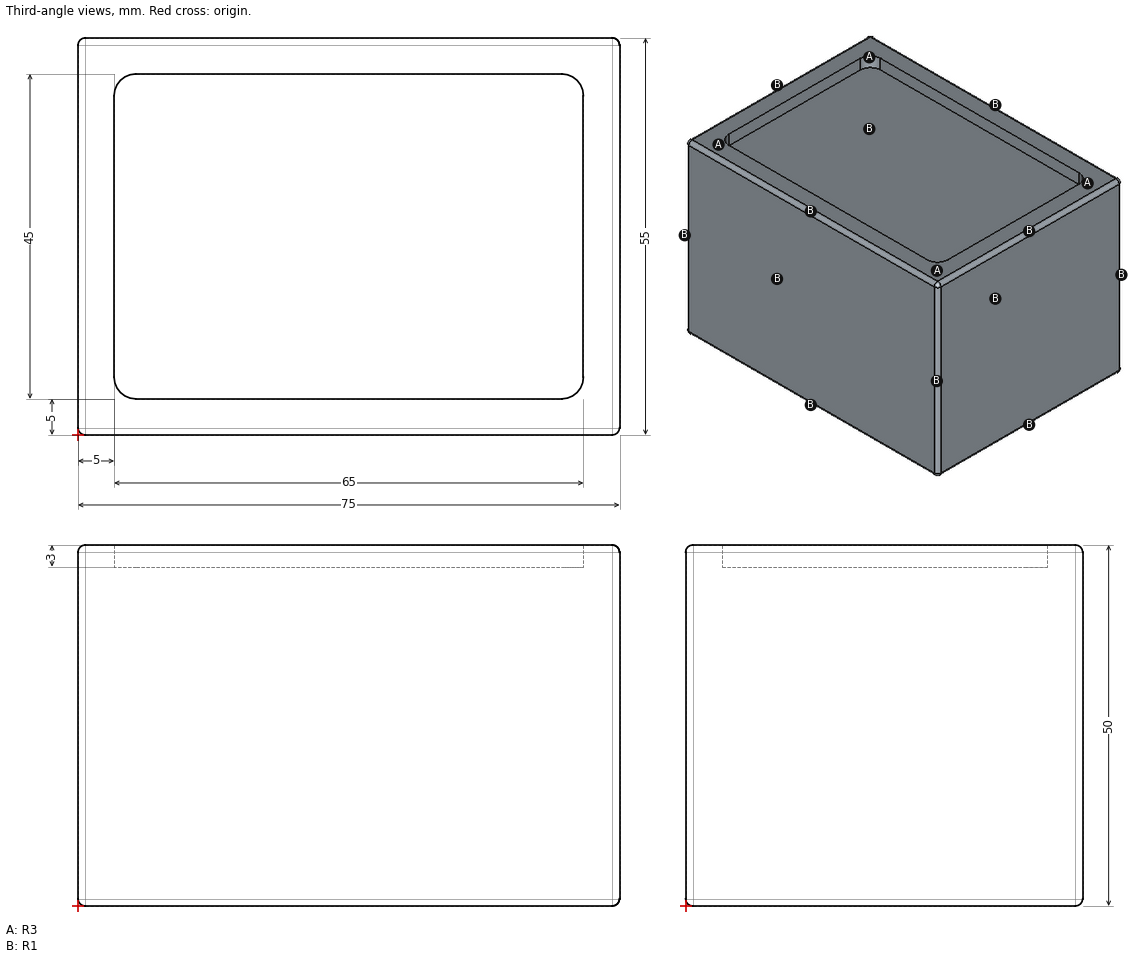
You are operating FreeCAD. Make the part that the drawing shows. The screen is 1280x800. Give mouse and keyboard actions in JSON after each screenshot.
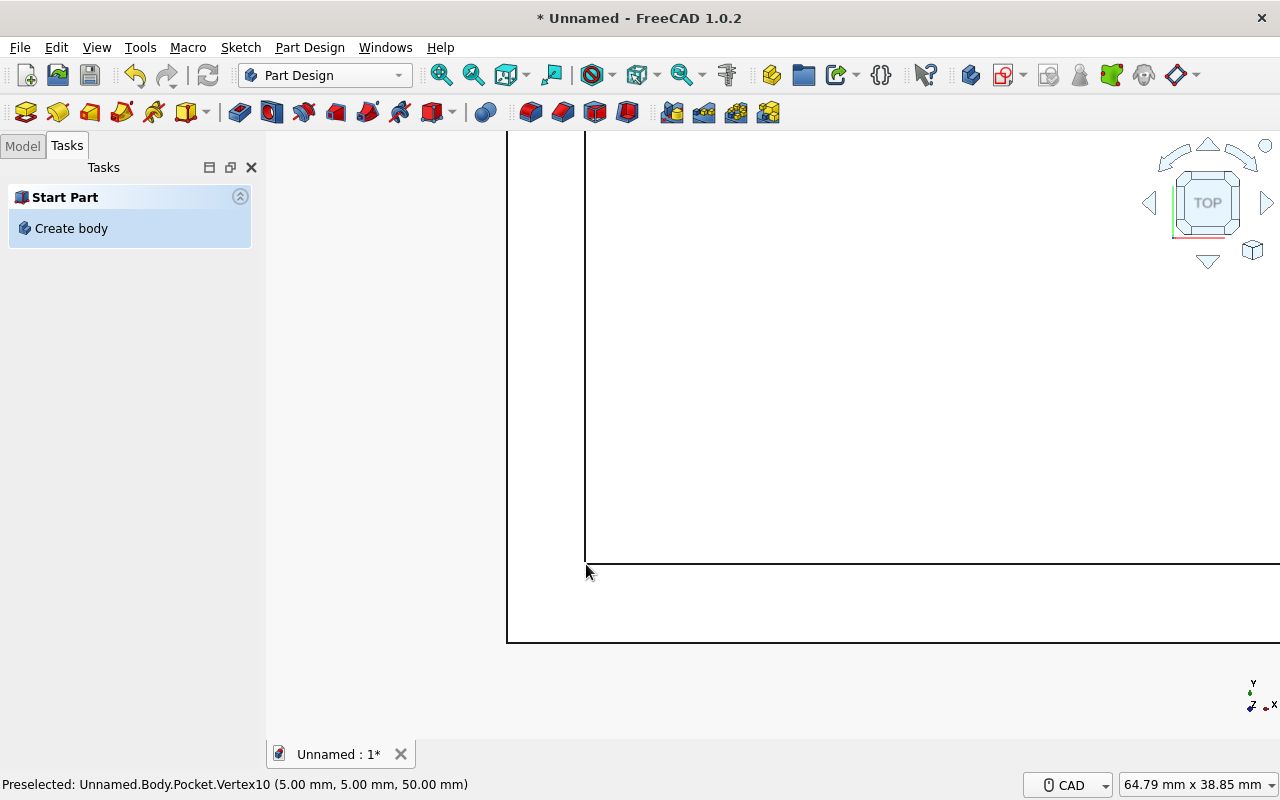
{"action": "left_click", "coordinate": [442, 76]}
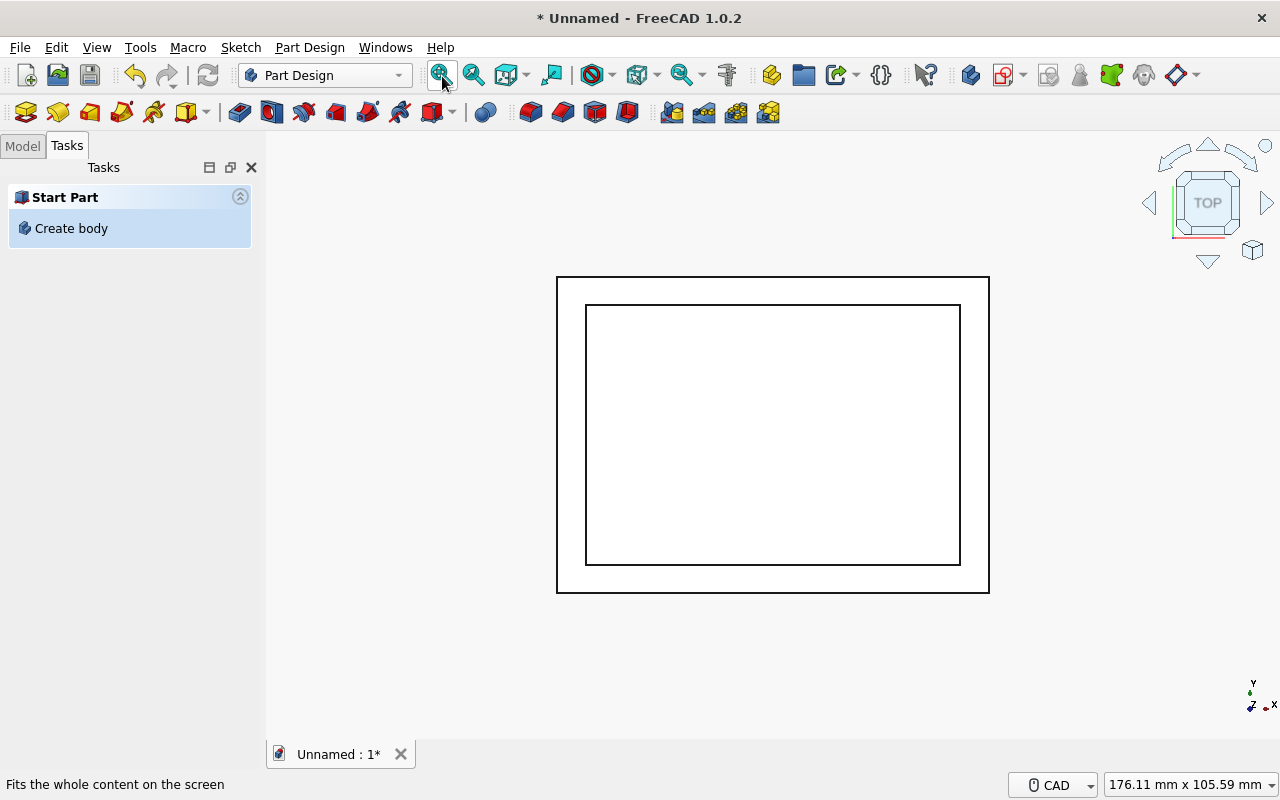
{"action": "key", "text": "1"}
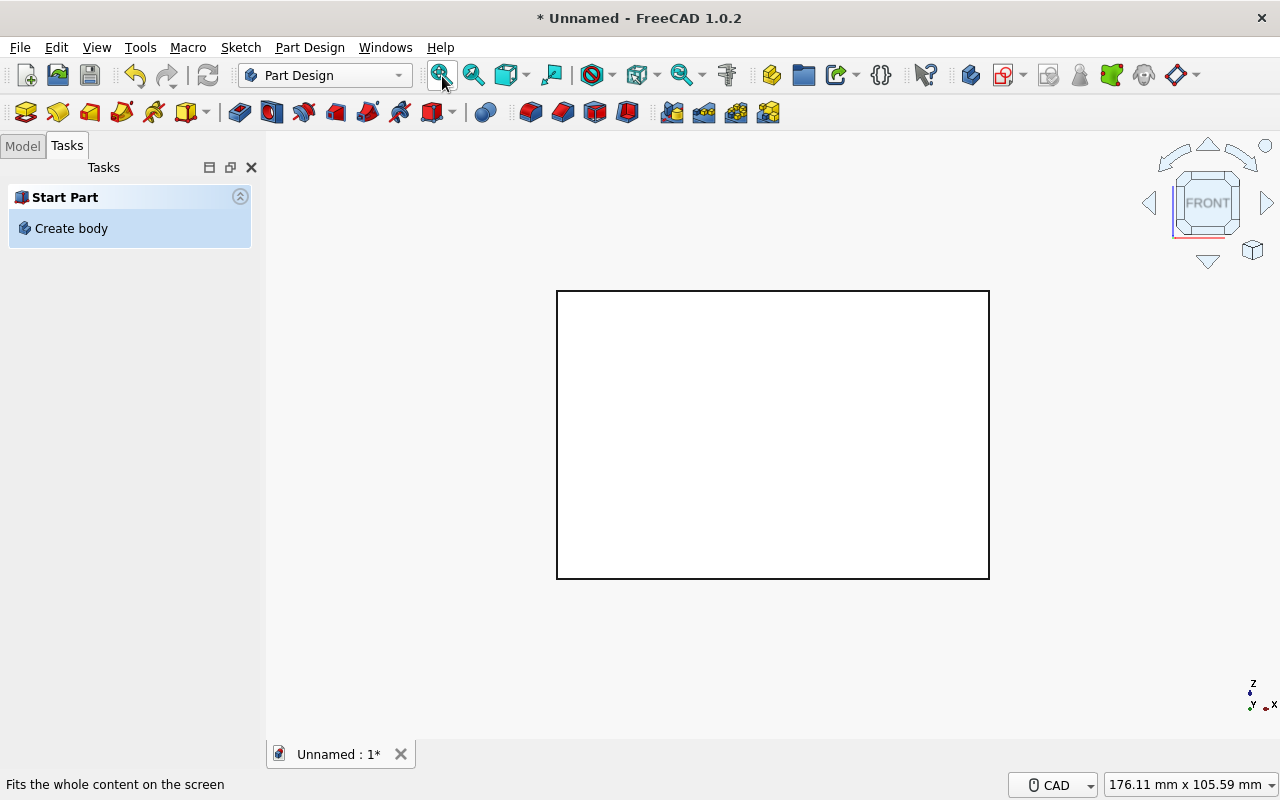
{"action": "scroll", "coordinate": [586, 299], "scroll_direction": "up", "scroll_amount": 5}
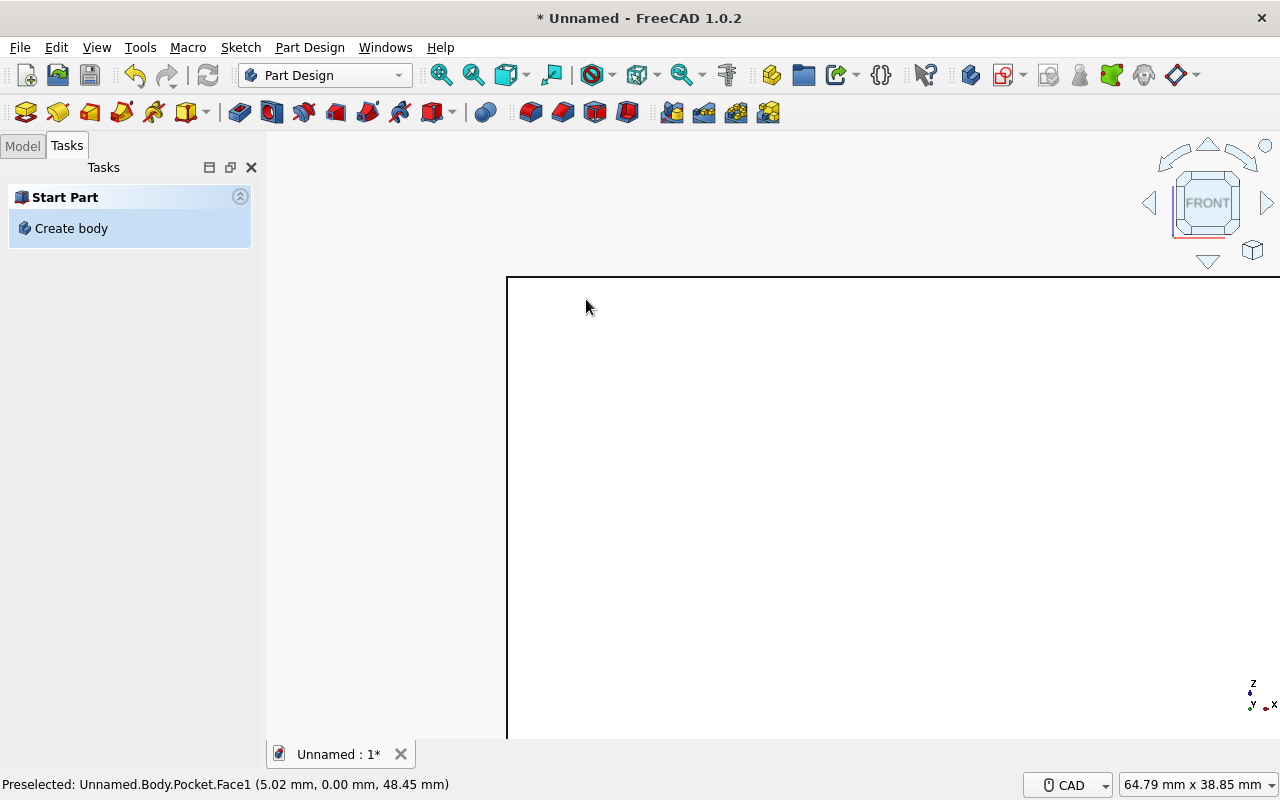
{"action": "left_click", "coordinate": [442, 76]}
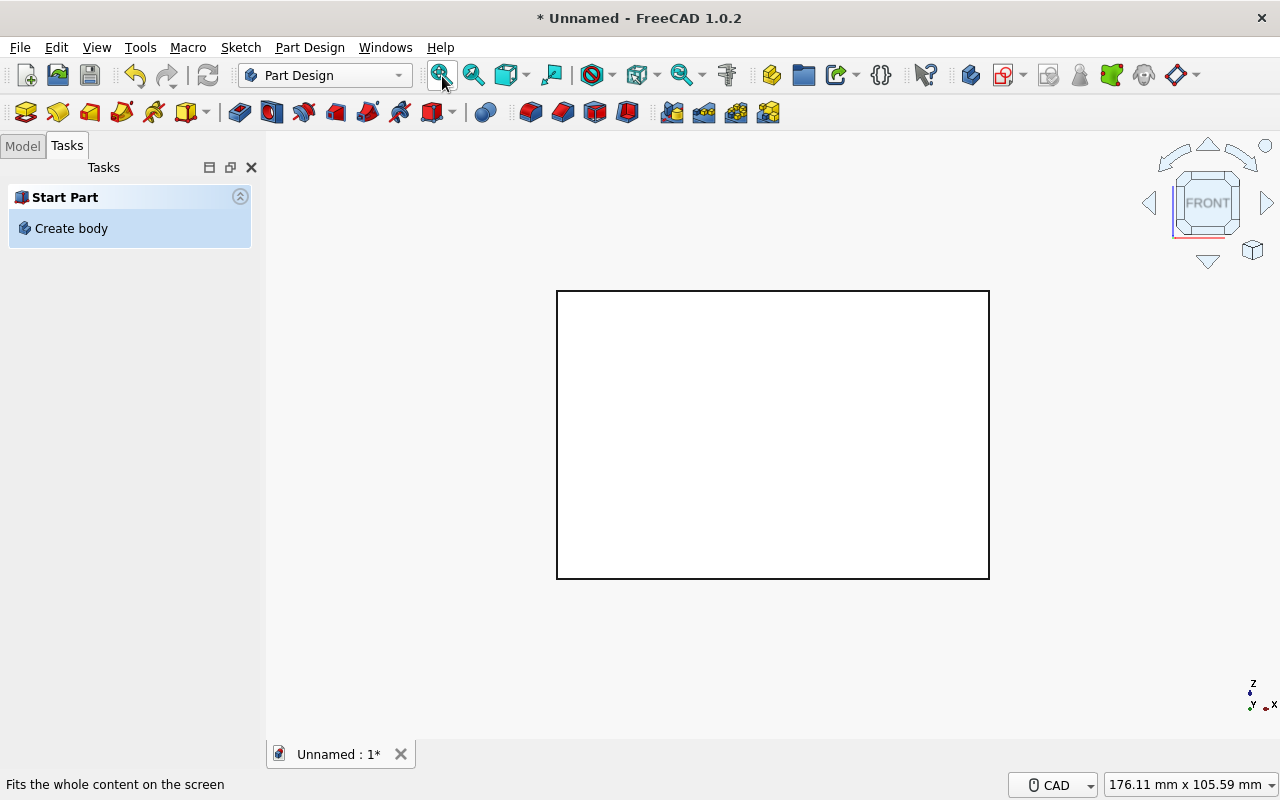
{"action": "key", "text": "3"}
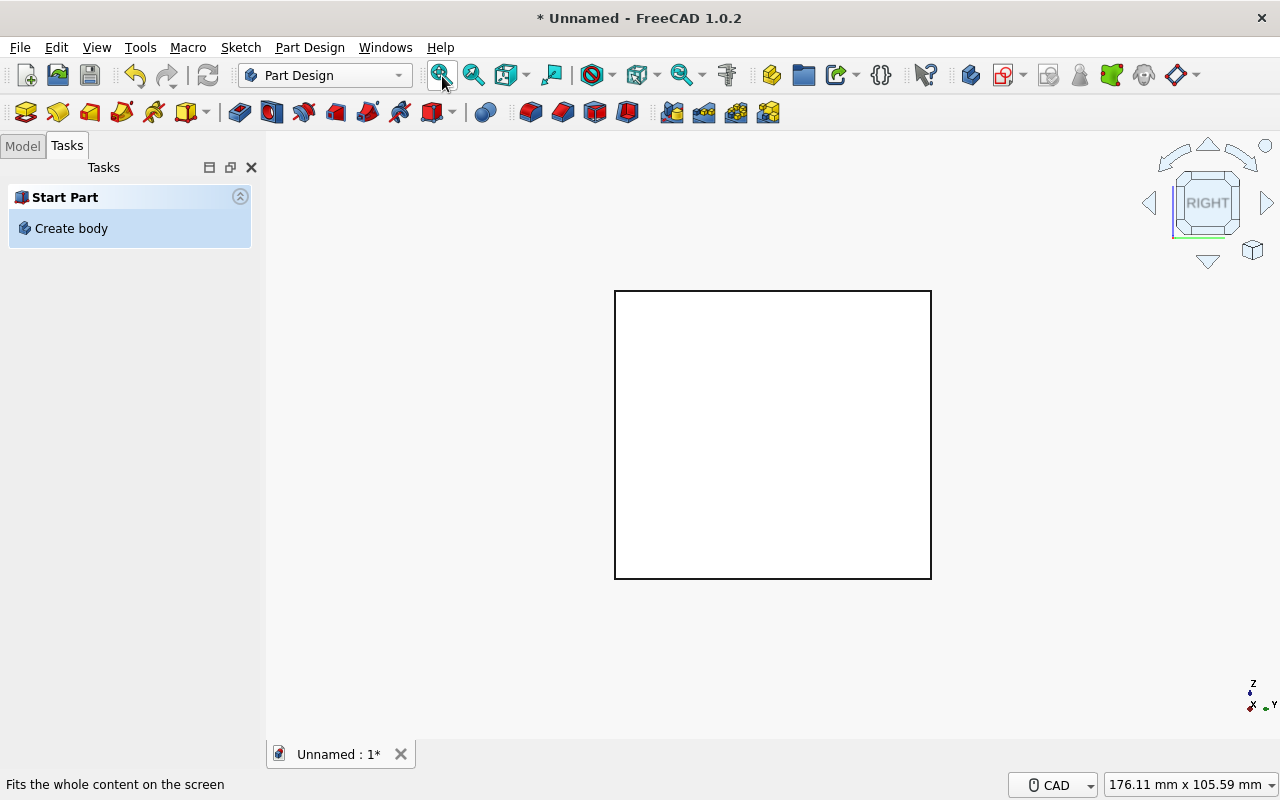
{"action": "scroll", "coordinate": [643, 299], "scroll_direction": "up", "scroll_amount": 5}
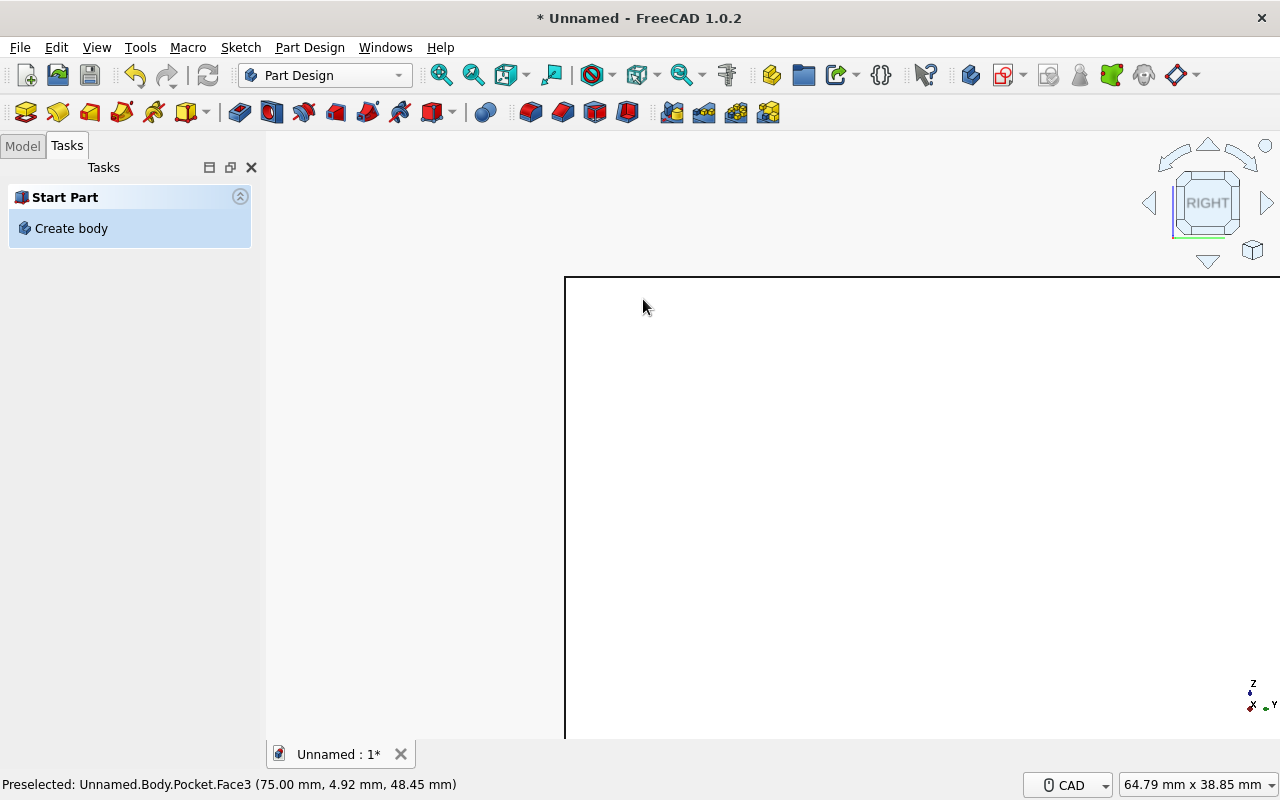
{"action": "left_click", "coordinate": [442, 76]}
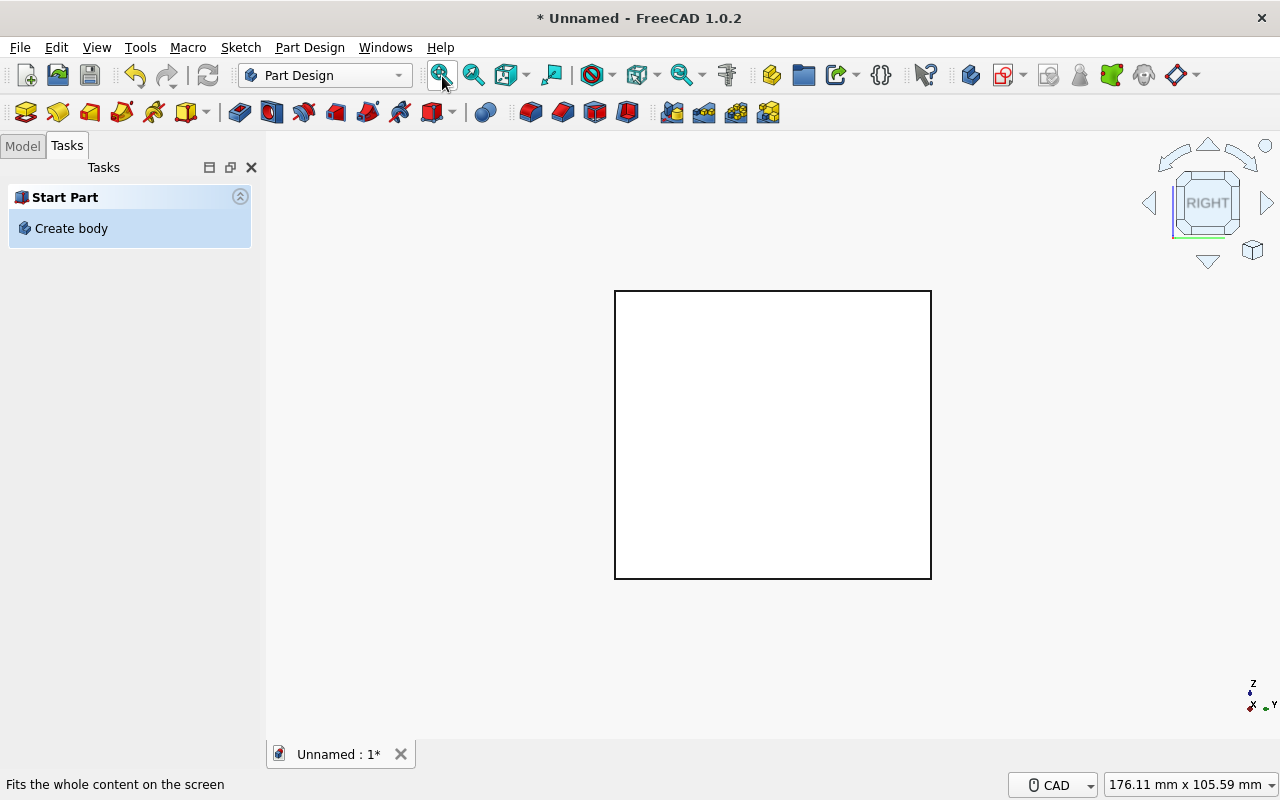
{"action": "key", "text": "5"}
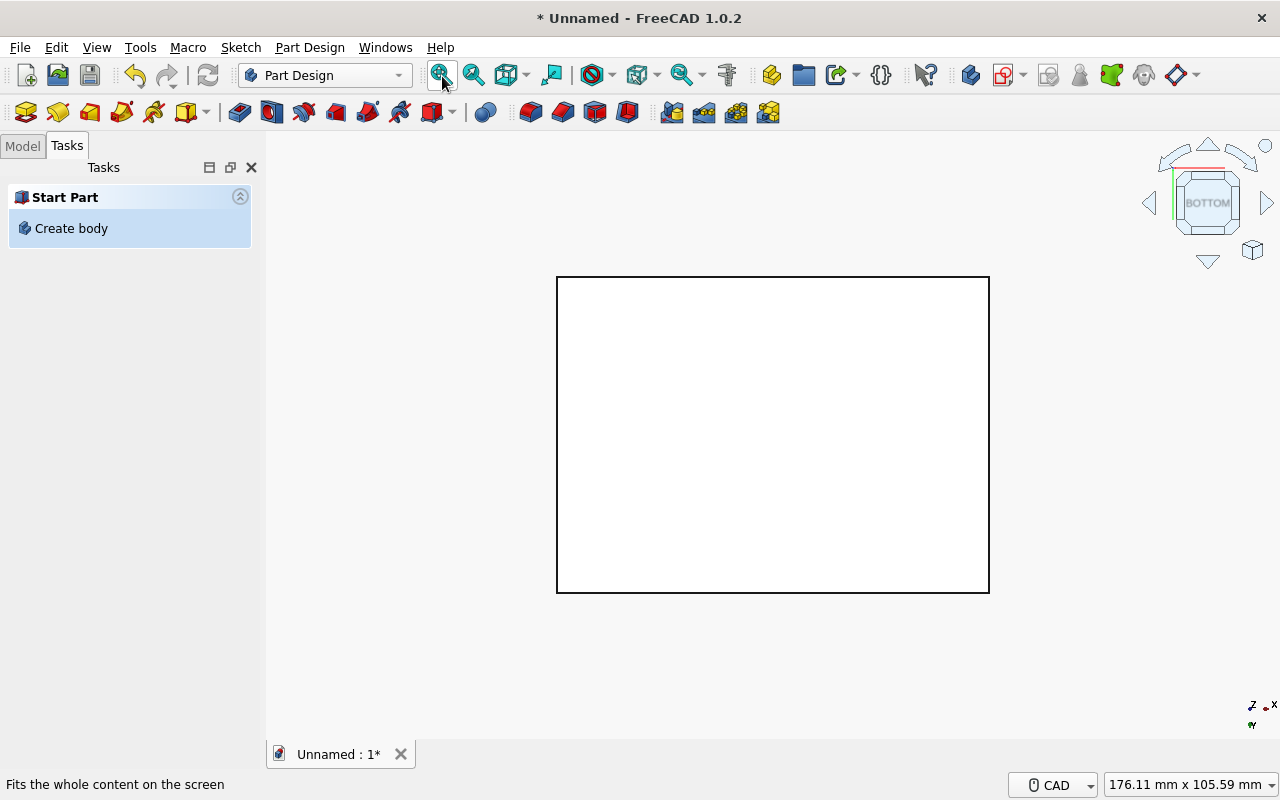
{"action": "scroll", "coordinate": [586, 304], "scroll_direction": "up", "scroll_amount": 5}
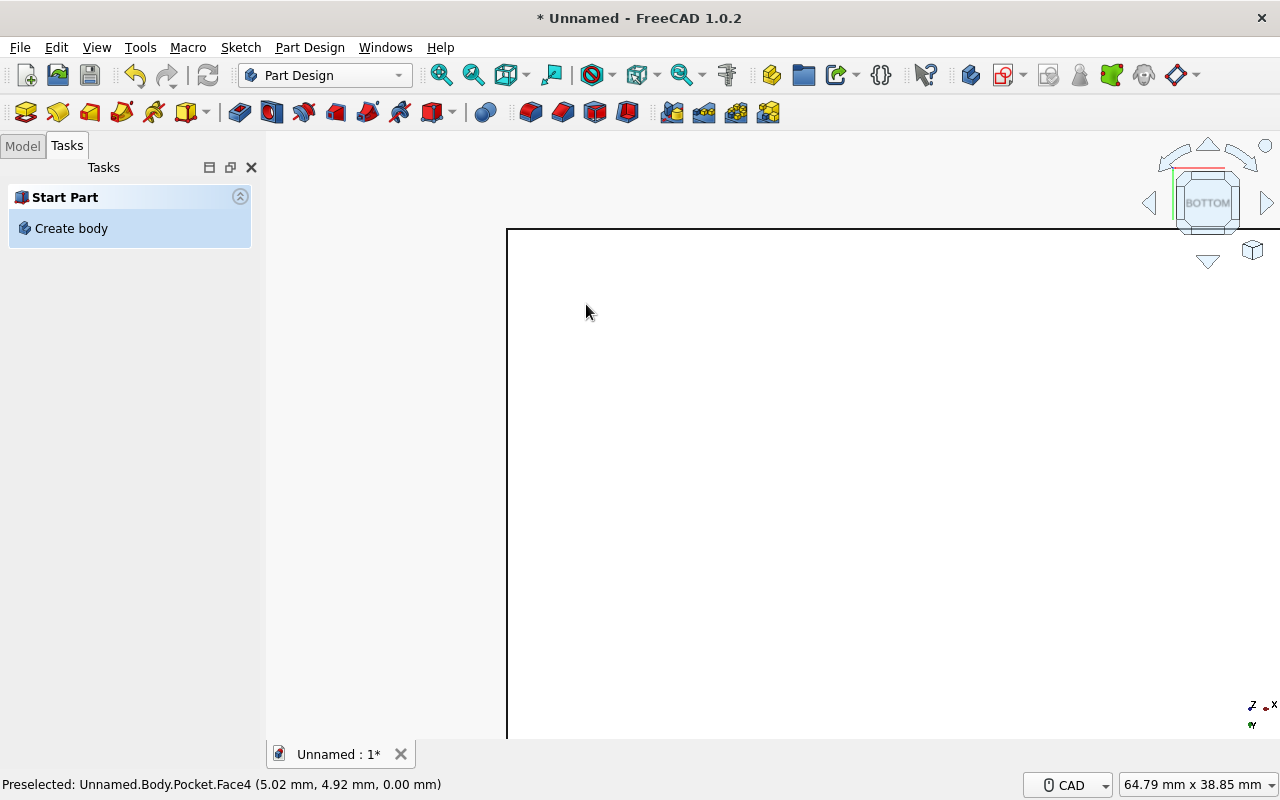
{"action": "left_click", "coordinate": [442, 76]}